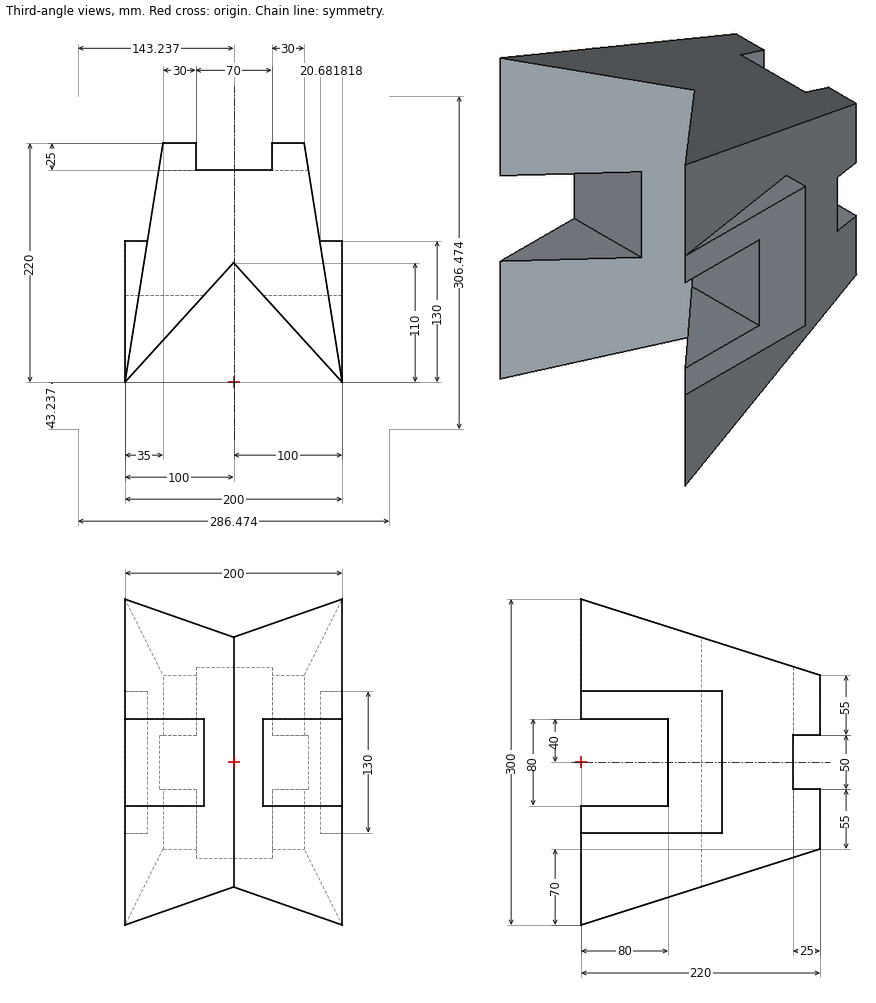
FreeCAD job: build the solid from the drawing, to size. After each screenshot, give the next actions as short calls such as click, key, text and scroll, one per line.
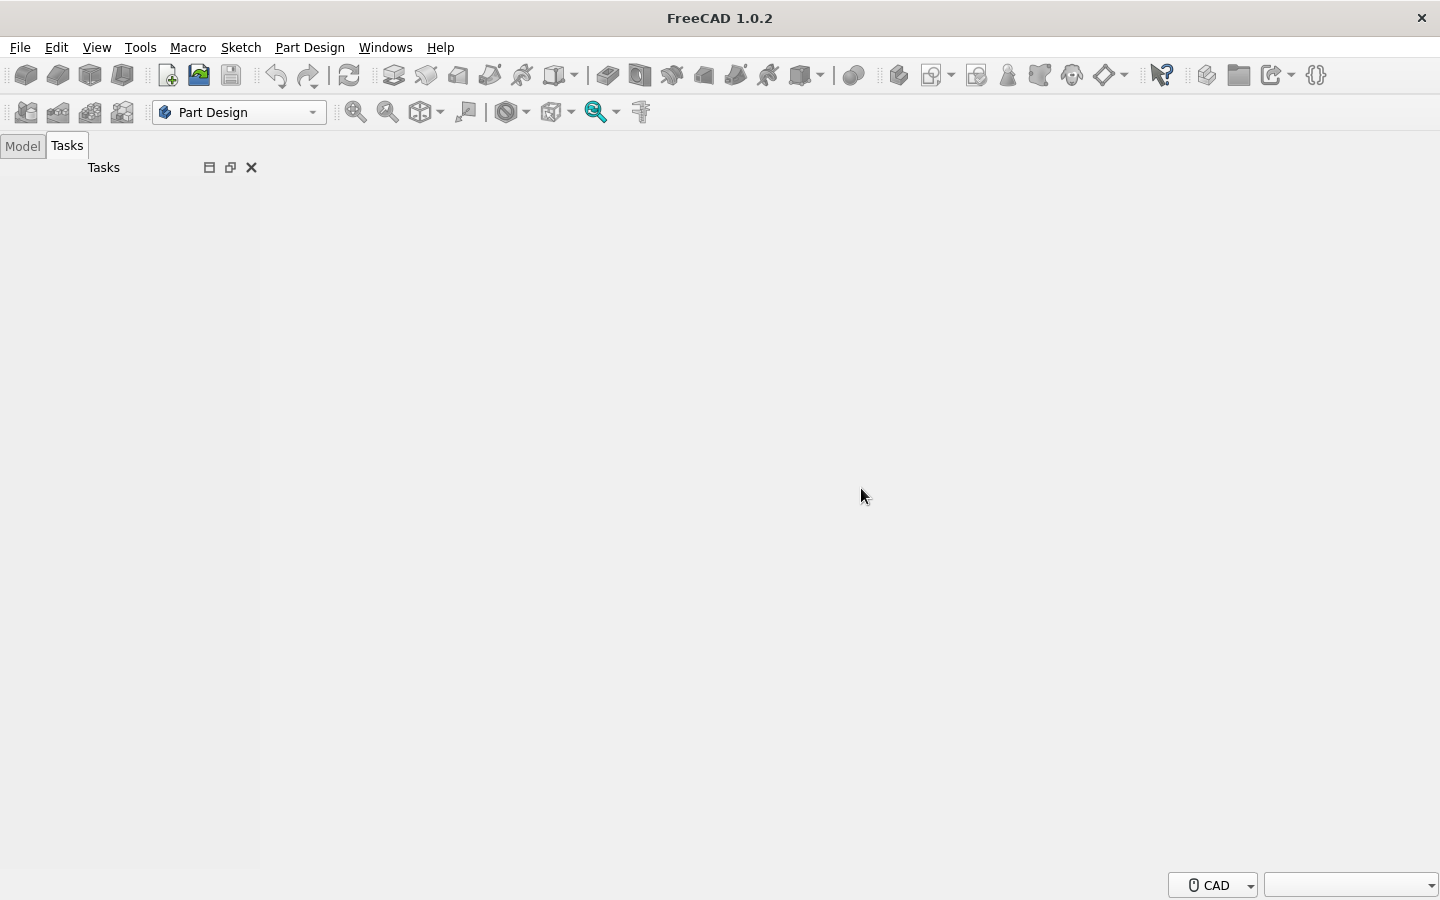
key(ctrl+n)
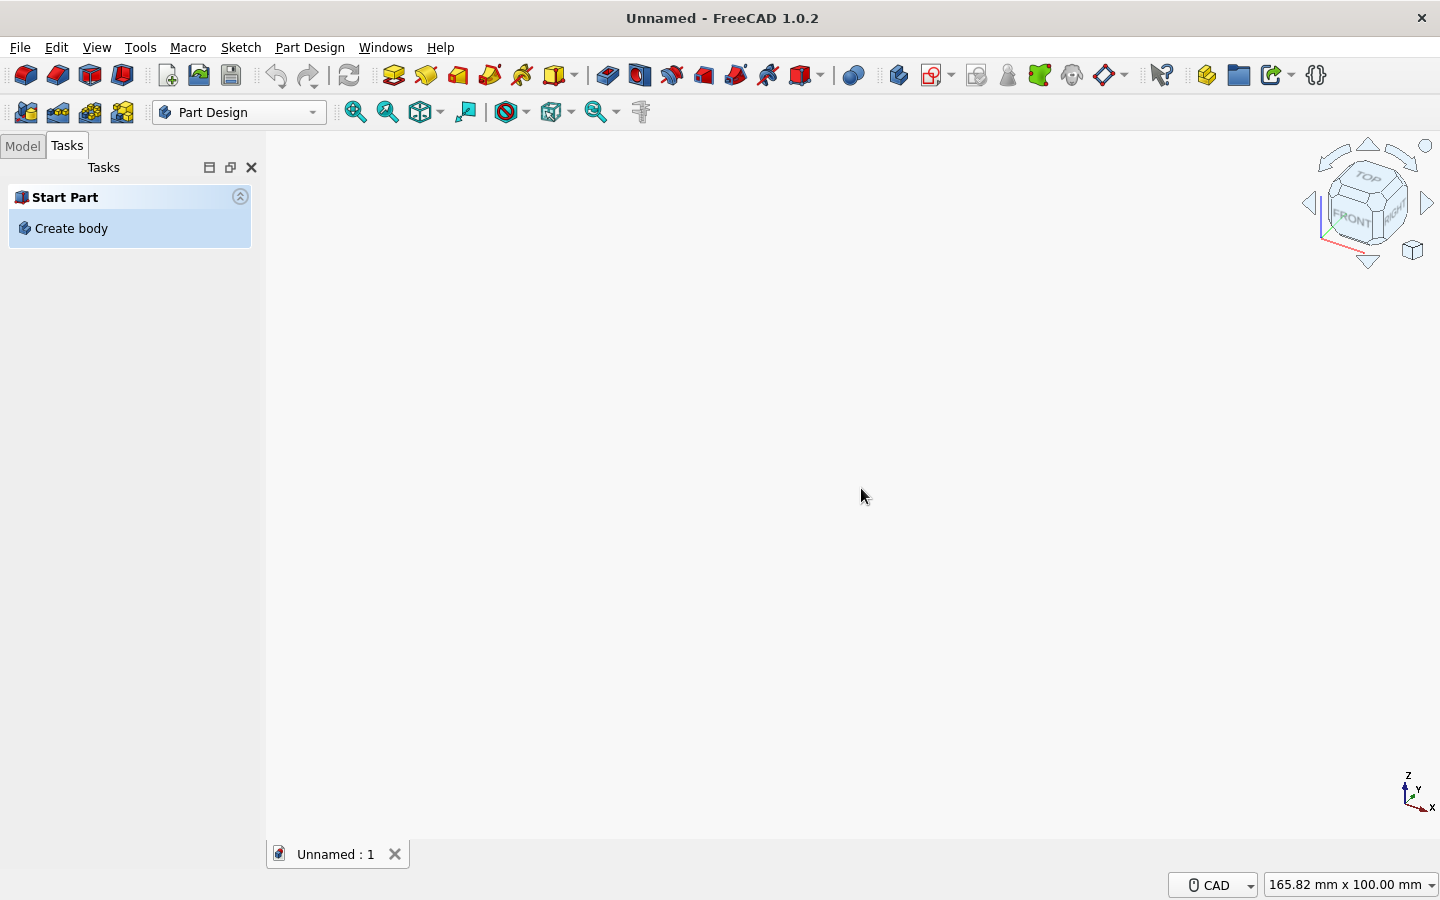
click(932, 76)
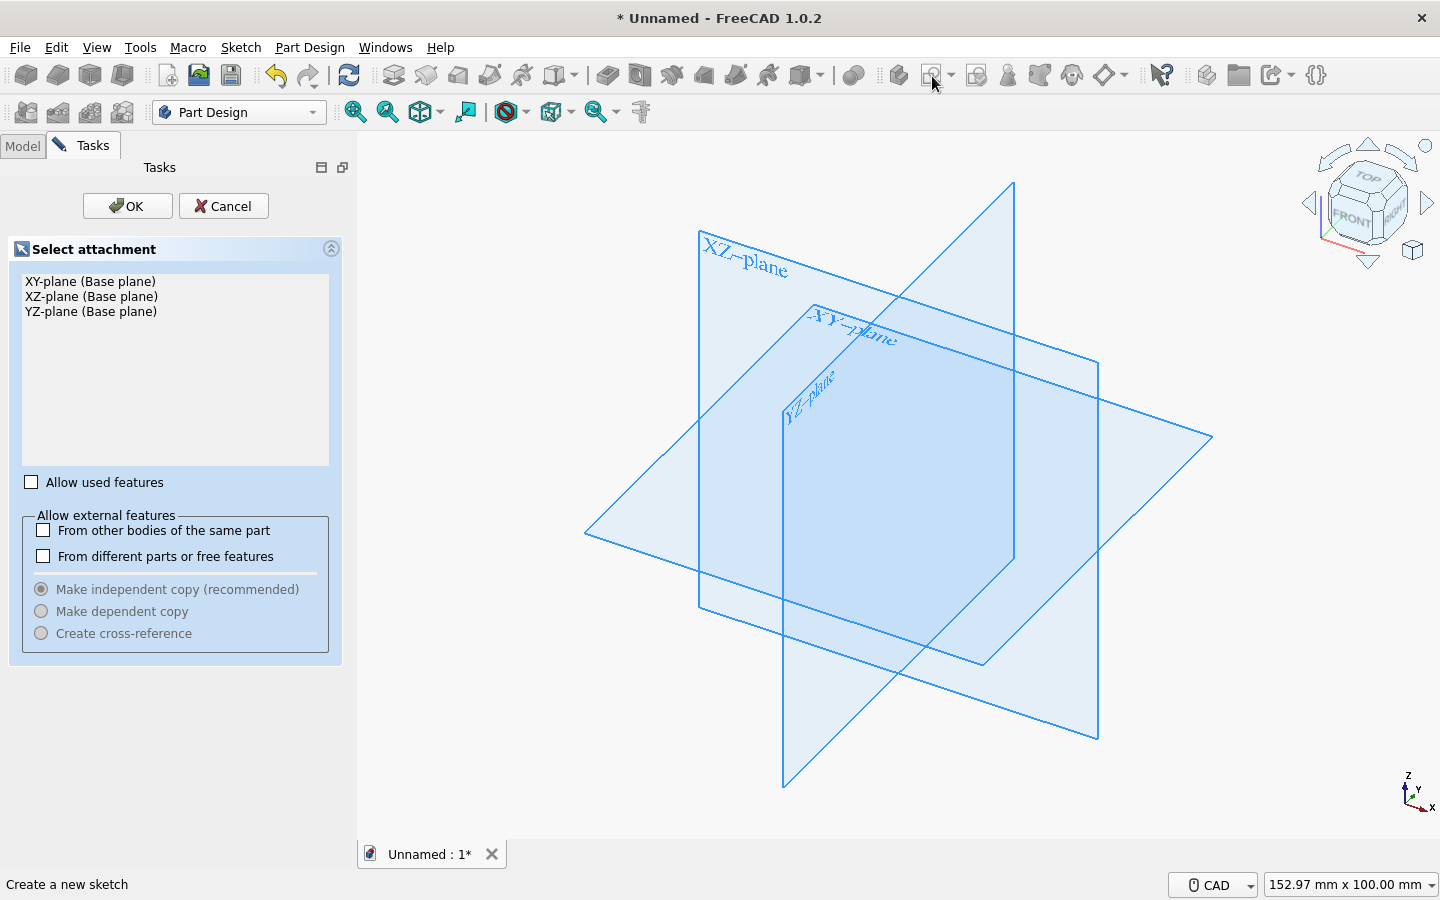
click(82, 312)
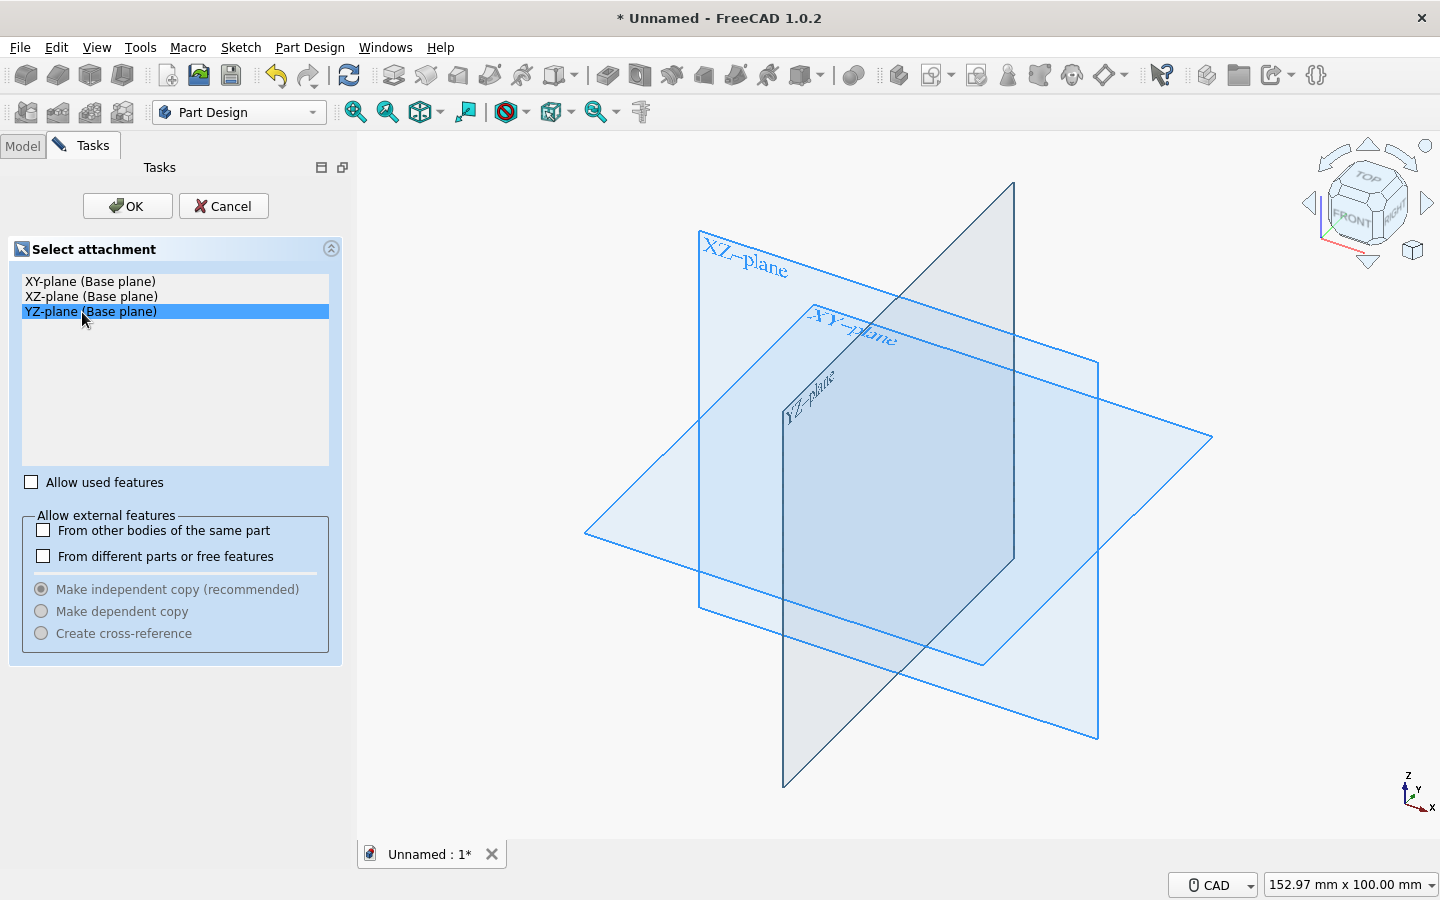
click(128, 206)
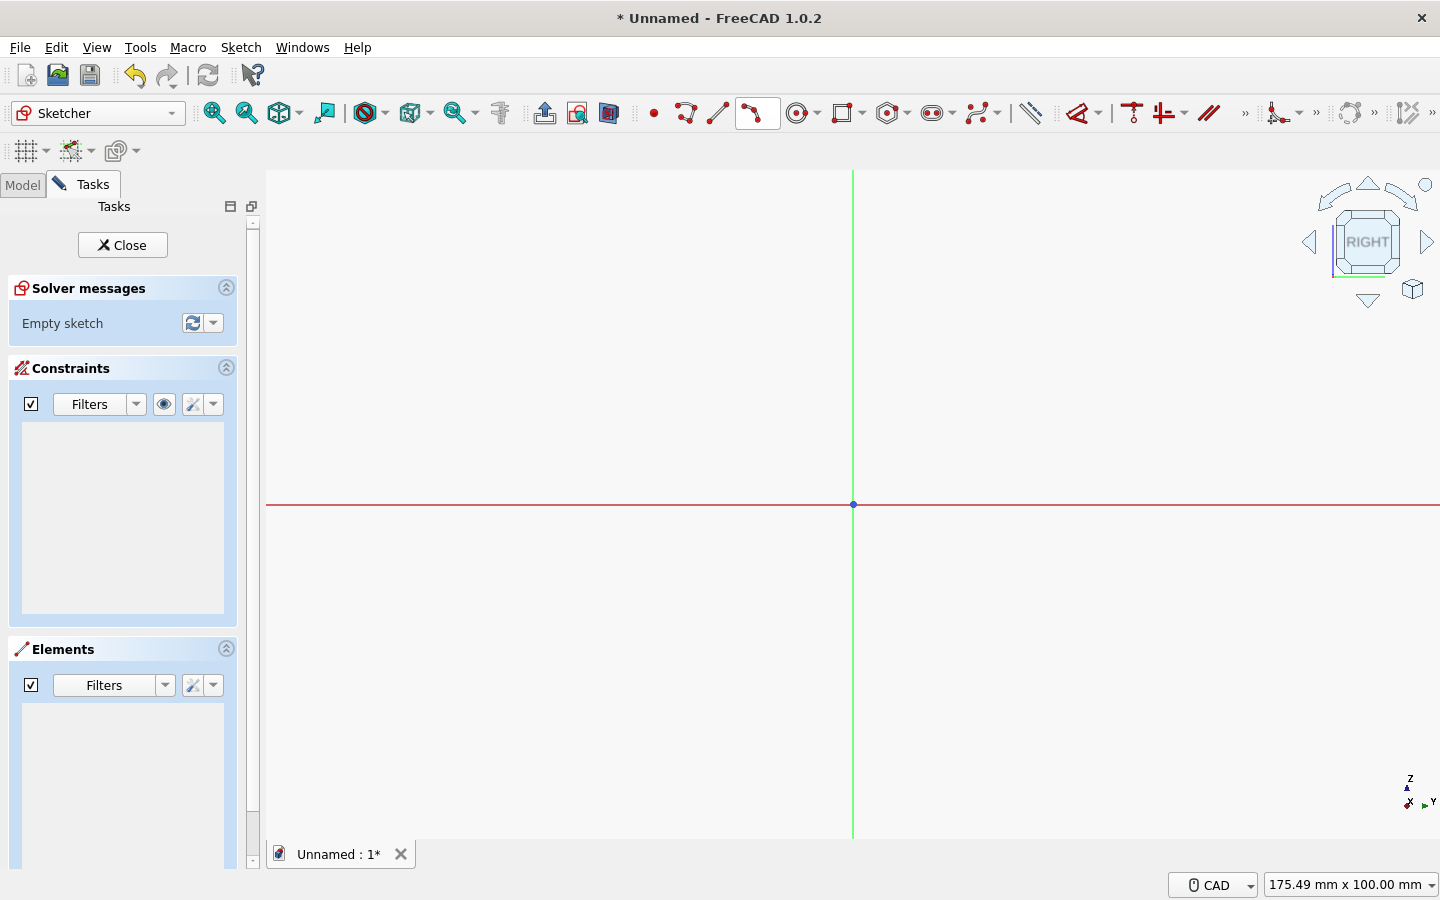
scroll(581, 504, down, 8)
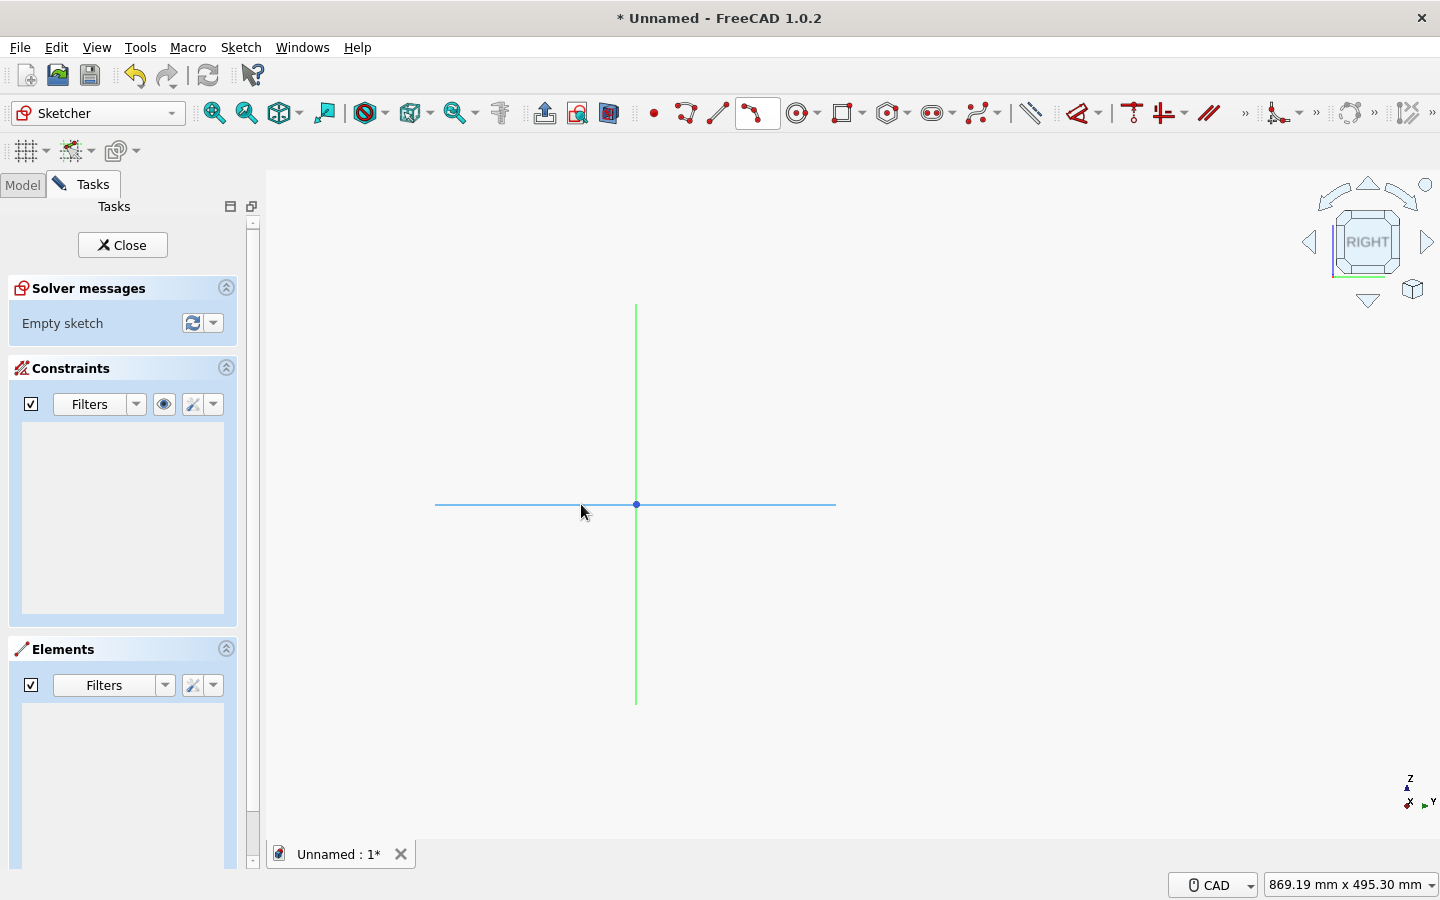
key(g)
key(m)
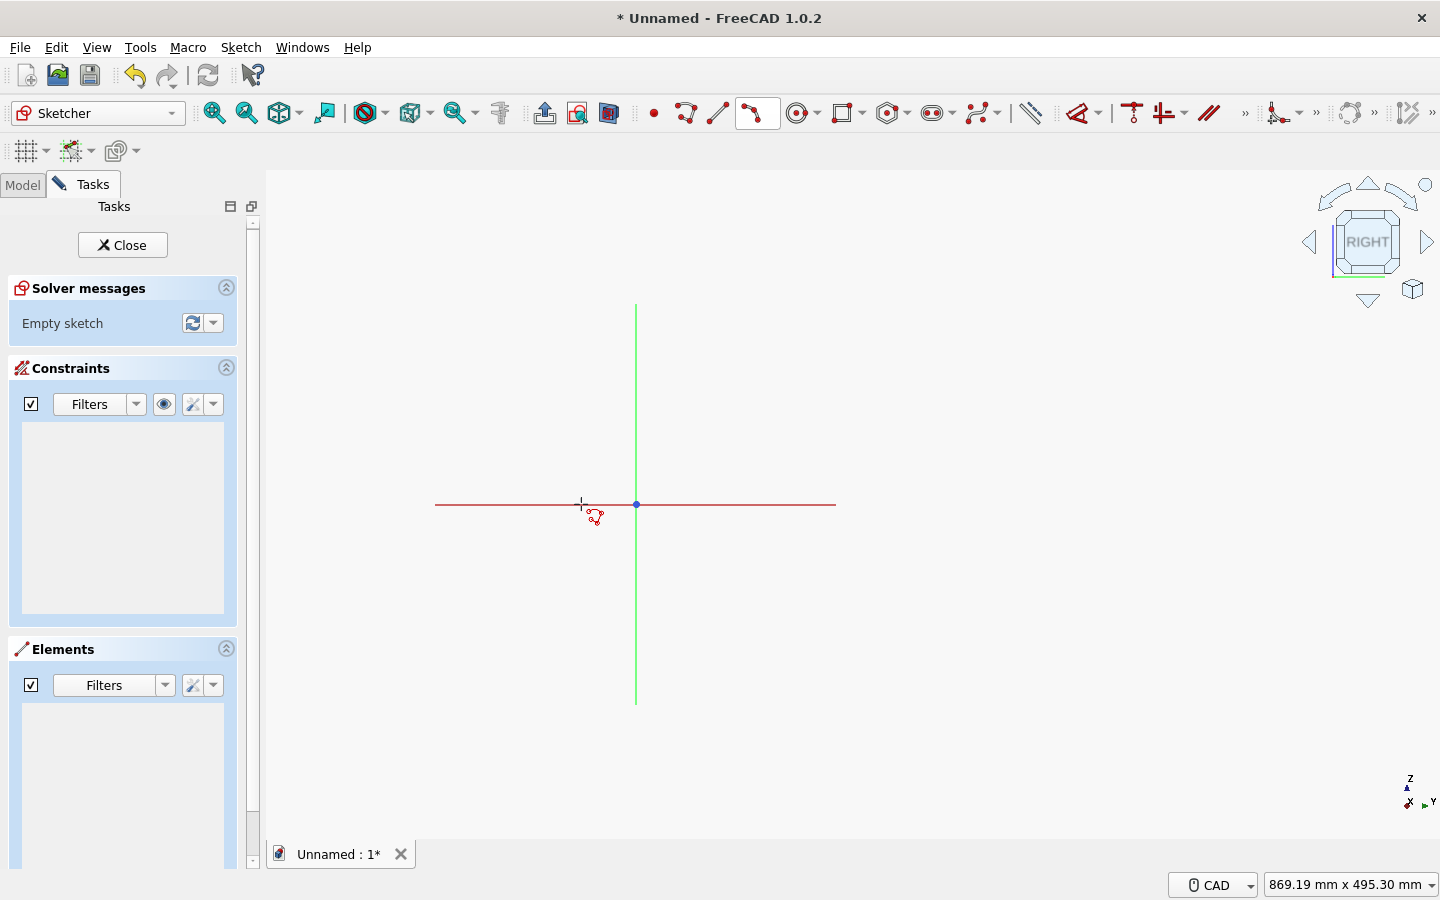
click(636, 302)
click(645, 707)
click(933, 613)
click(933, 538)
click(900, 538)
click(900, 471)
click(933, 471)
click(933, 396)
click(636, 303)
key(Escape)
key(Escape)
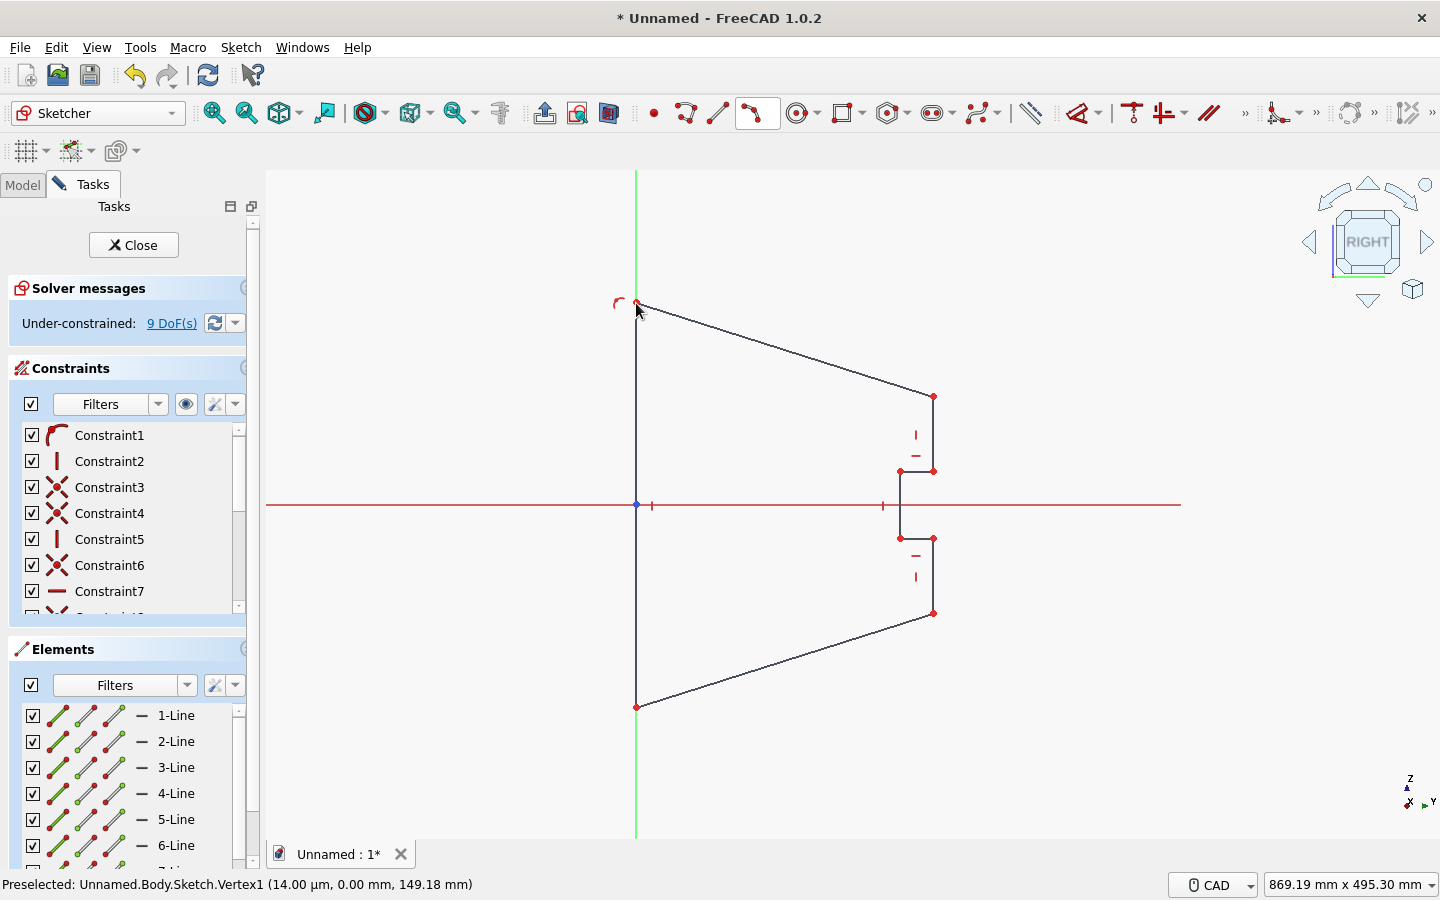
click(933, 539)